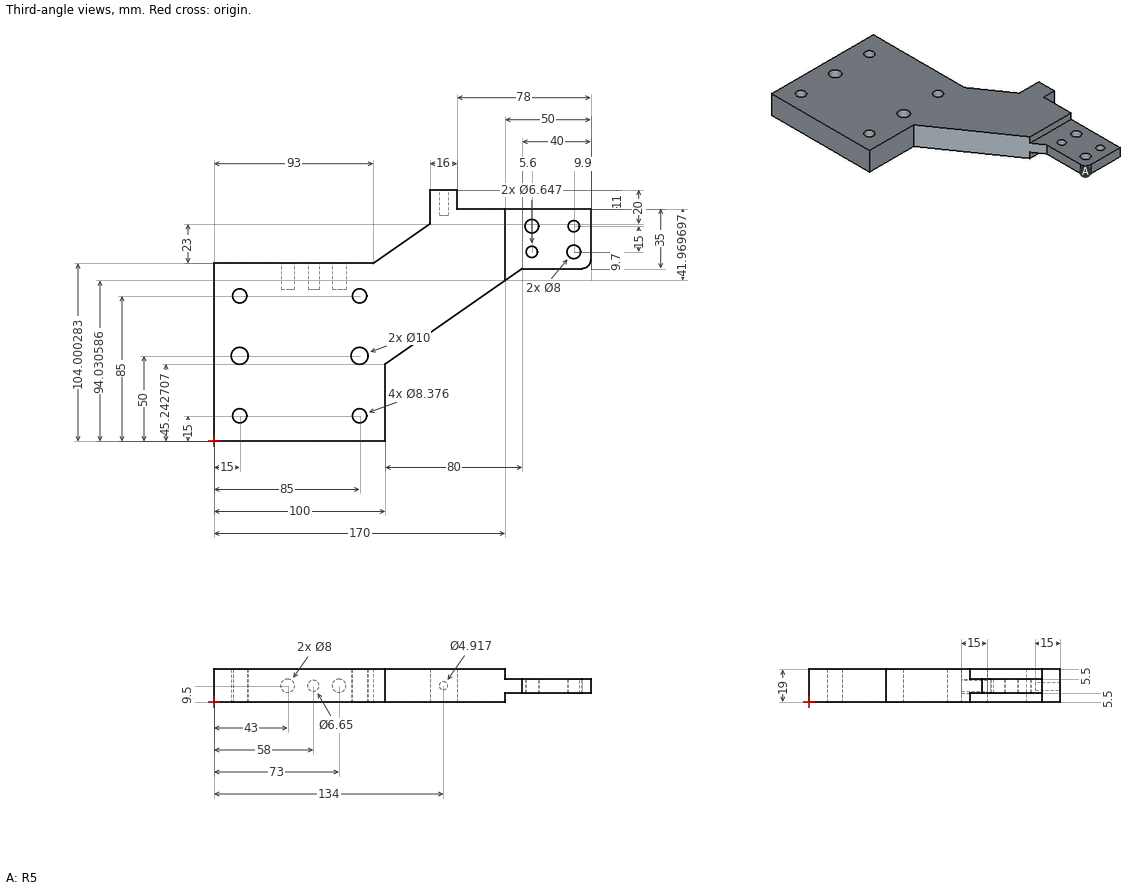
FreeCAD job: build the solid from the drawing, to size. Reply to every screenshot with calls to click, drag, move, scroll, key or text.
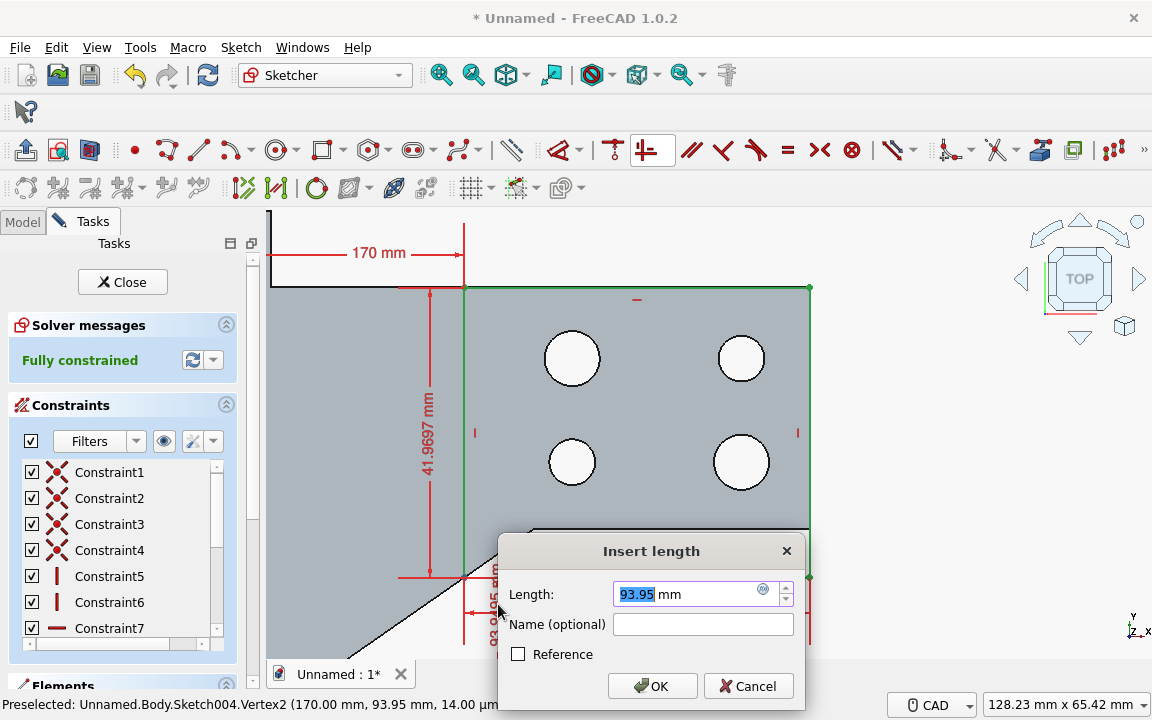
text(94.030586)
key(Return)
key(Escape)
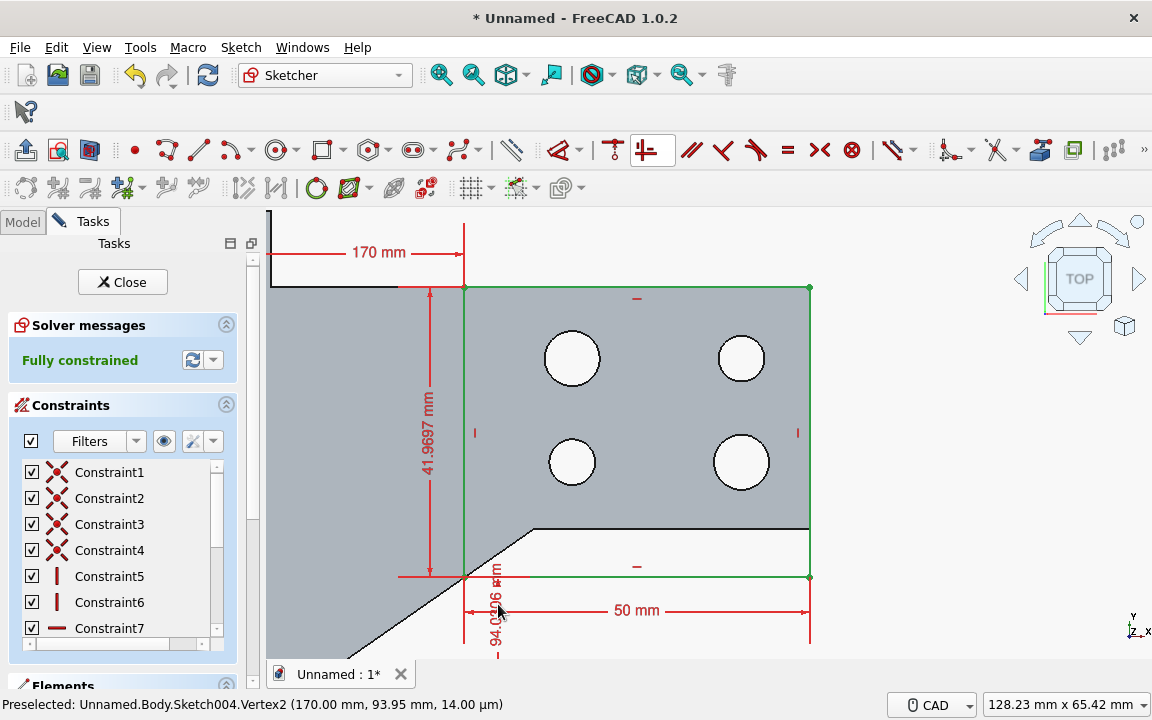
click(123, 282)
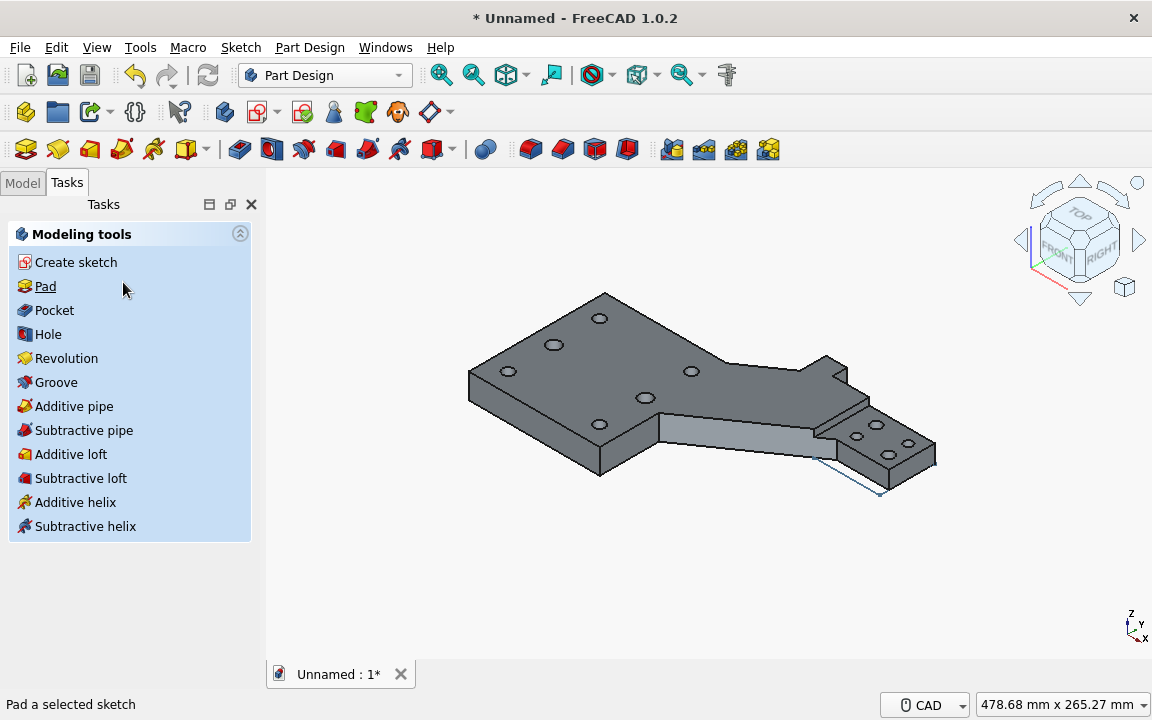
click(240, 150)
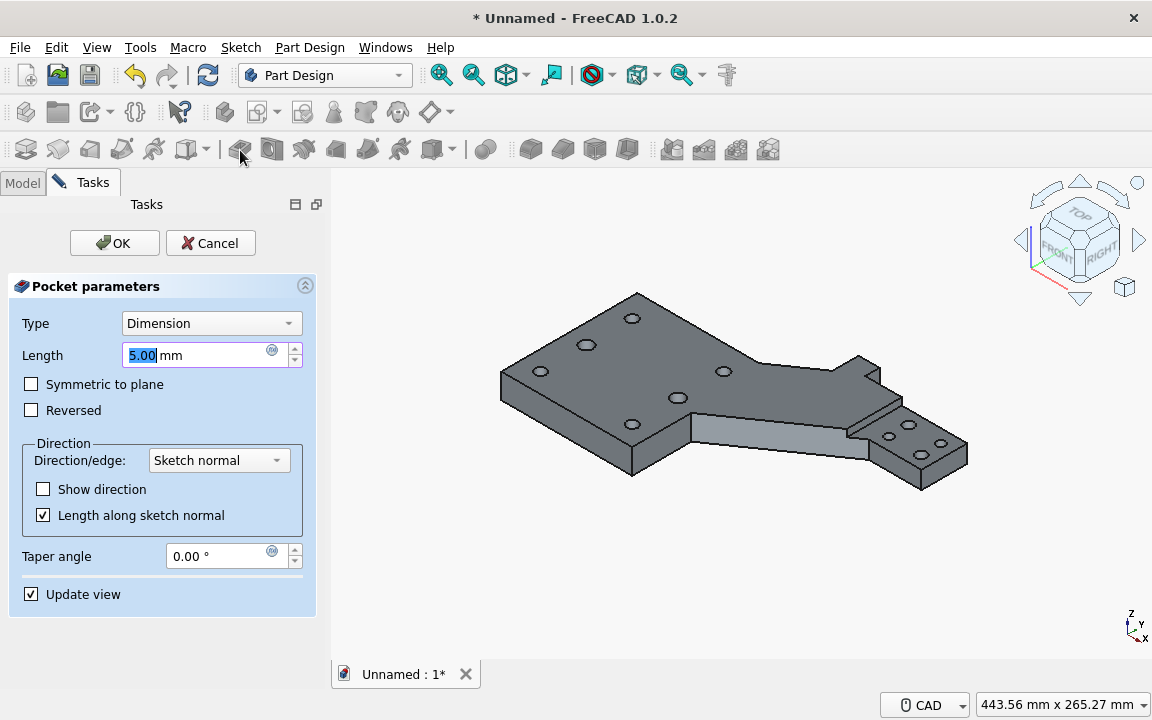
text(5.5)
key(Tab)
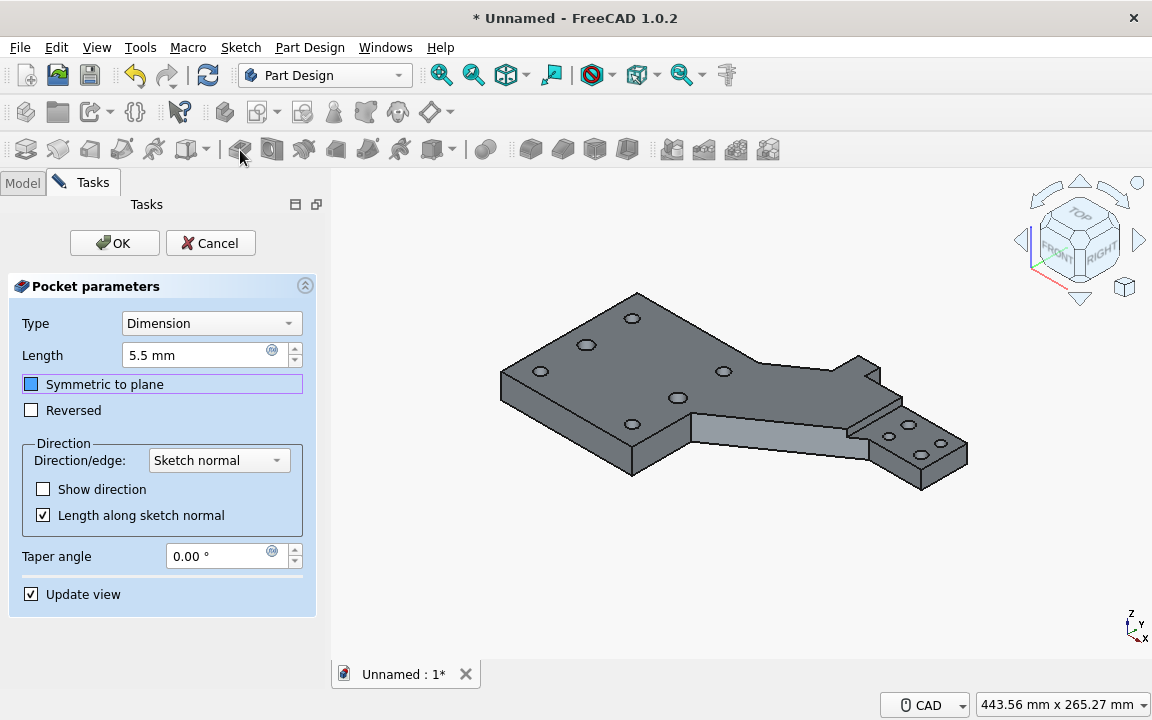
click(30, 410)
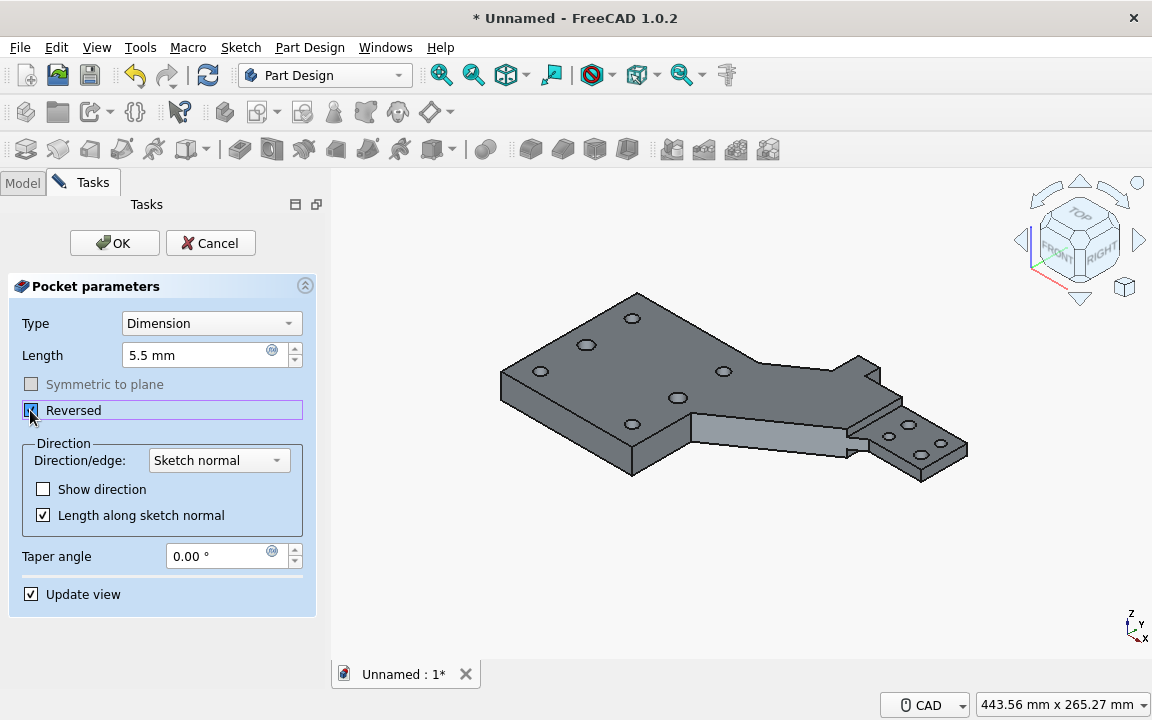
click(115, 243)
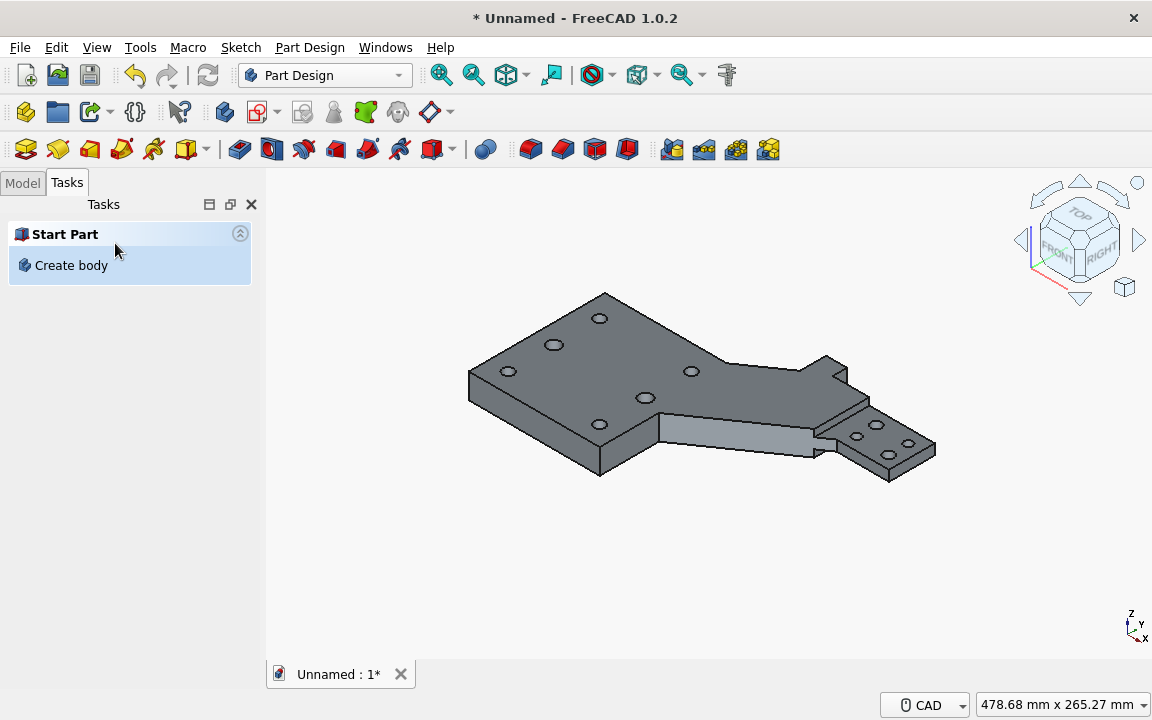
click(889, 475)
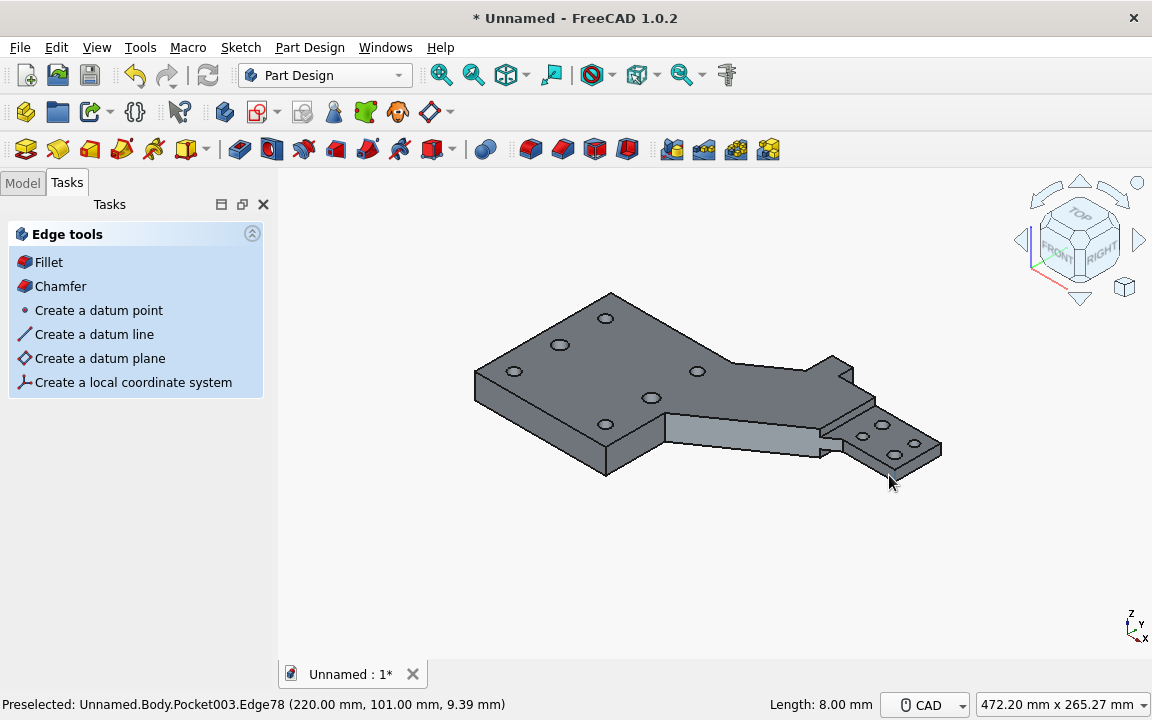
click(532, 150)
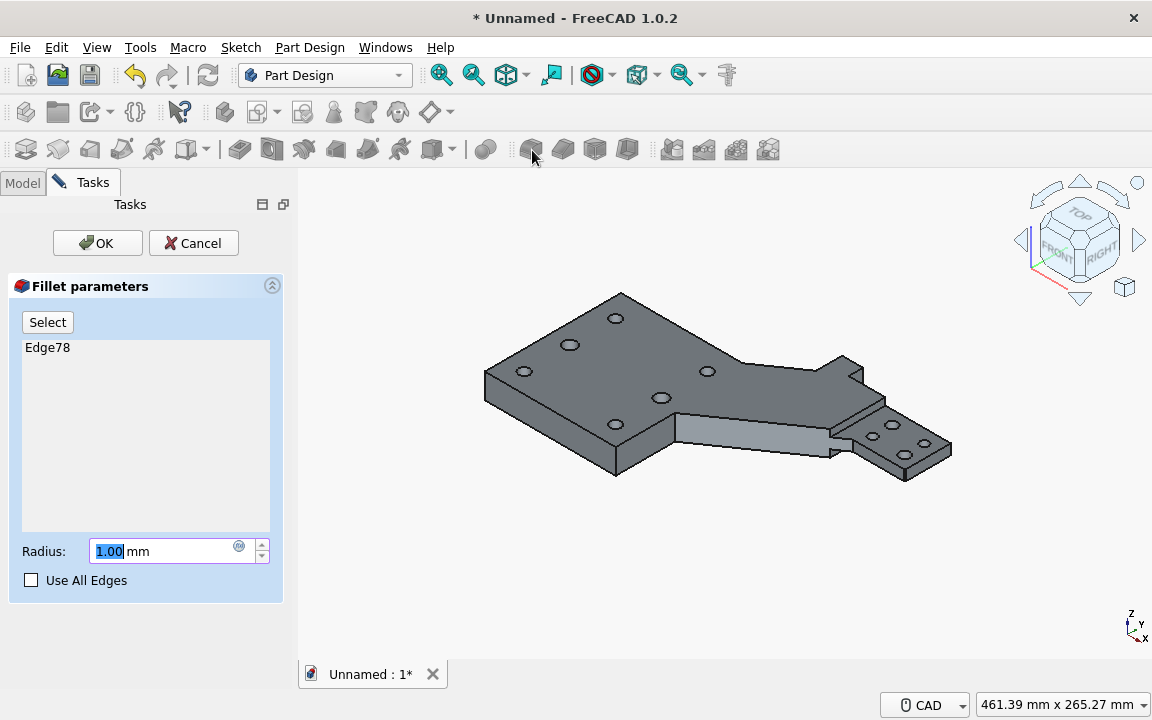
text(5)
key(Tab)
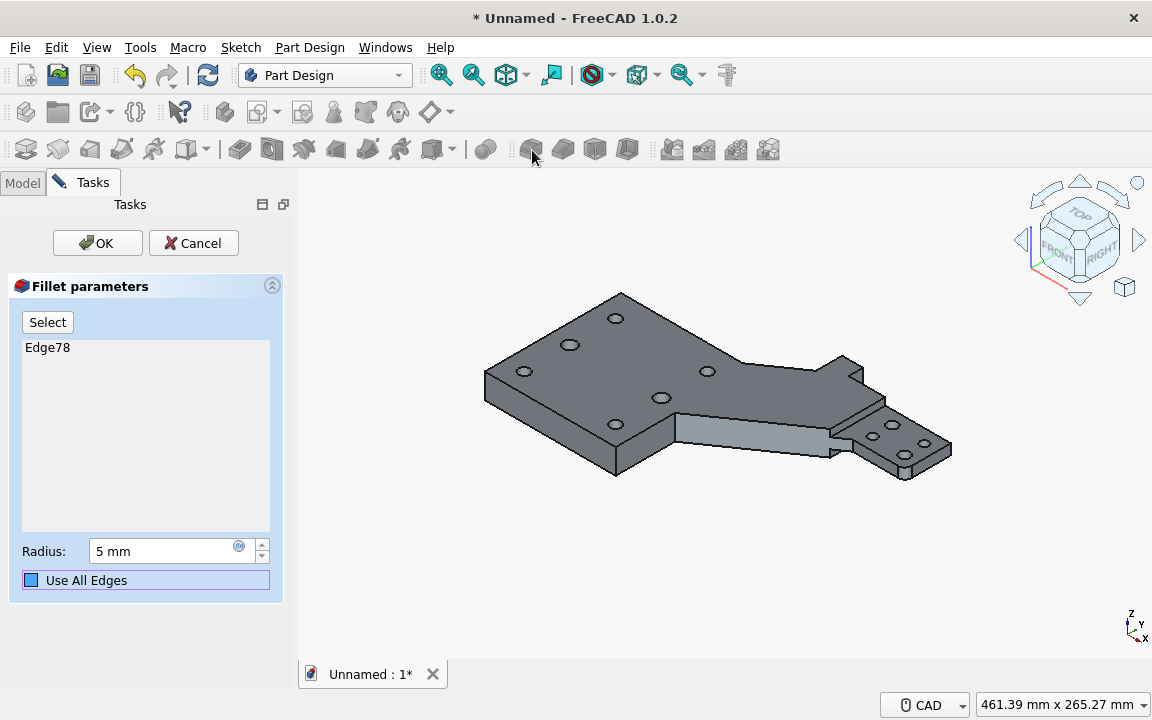
click(98, 243)